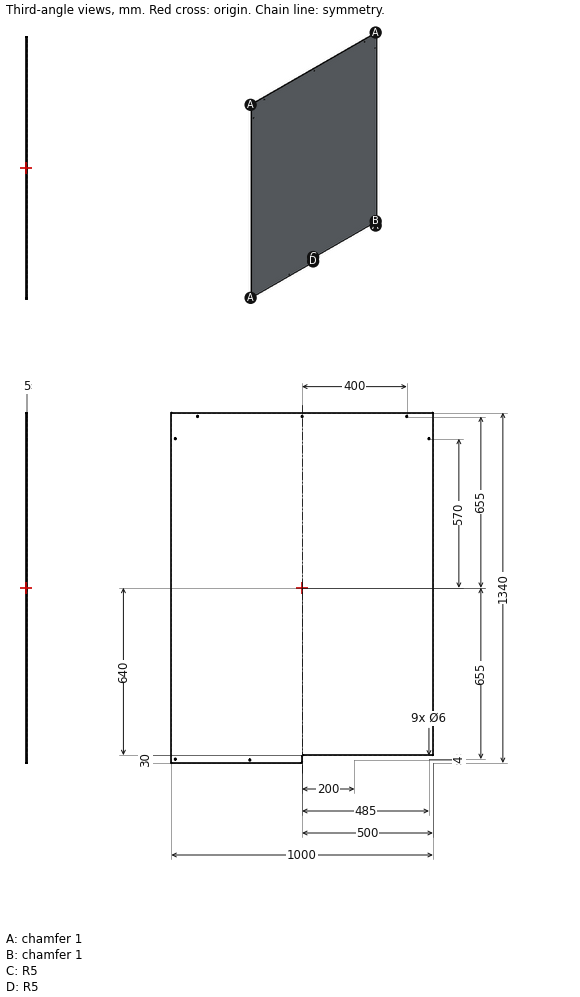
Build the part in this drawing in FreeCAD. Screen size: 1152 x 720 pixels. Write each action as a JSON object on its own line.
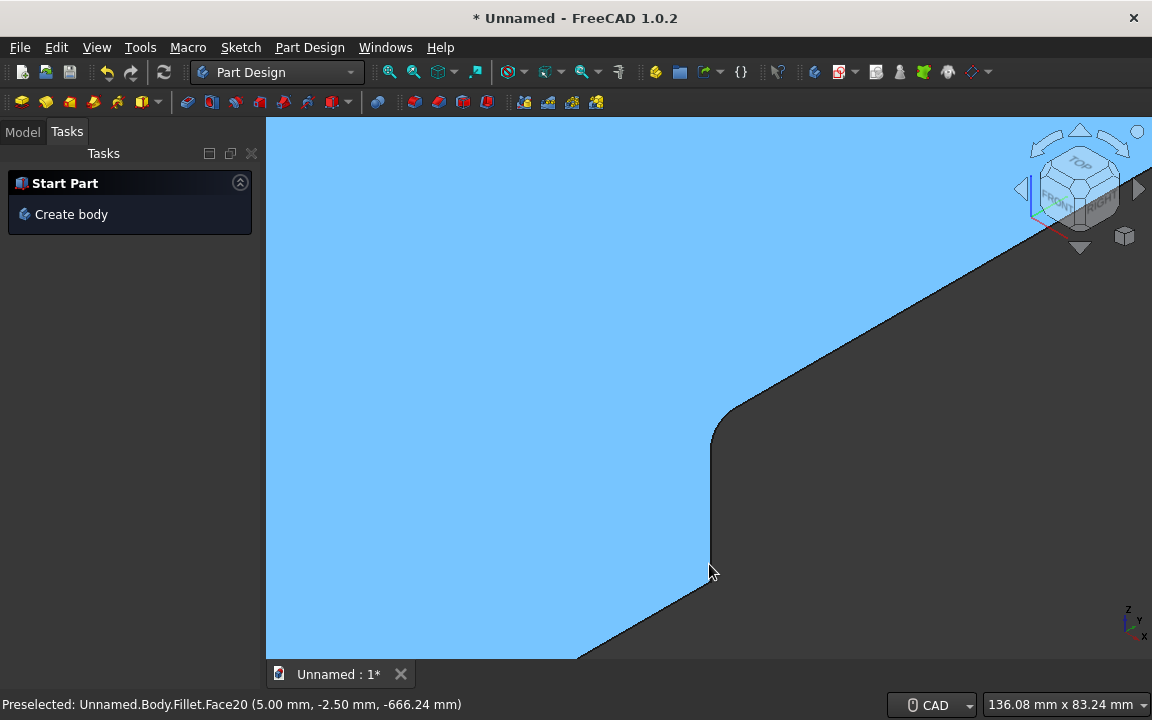
{"action": "left_click", "coordinate": [390, 72]}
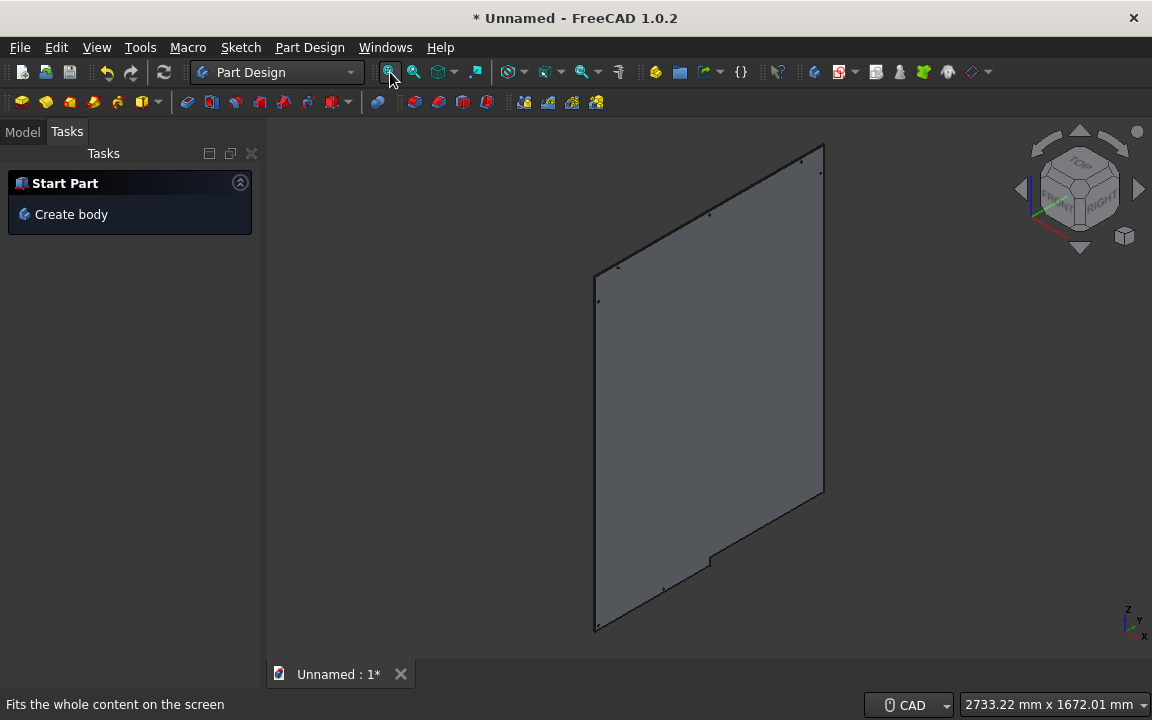
{"action": "key", "text": "1"}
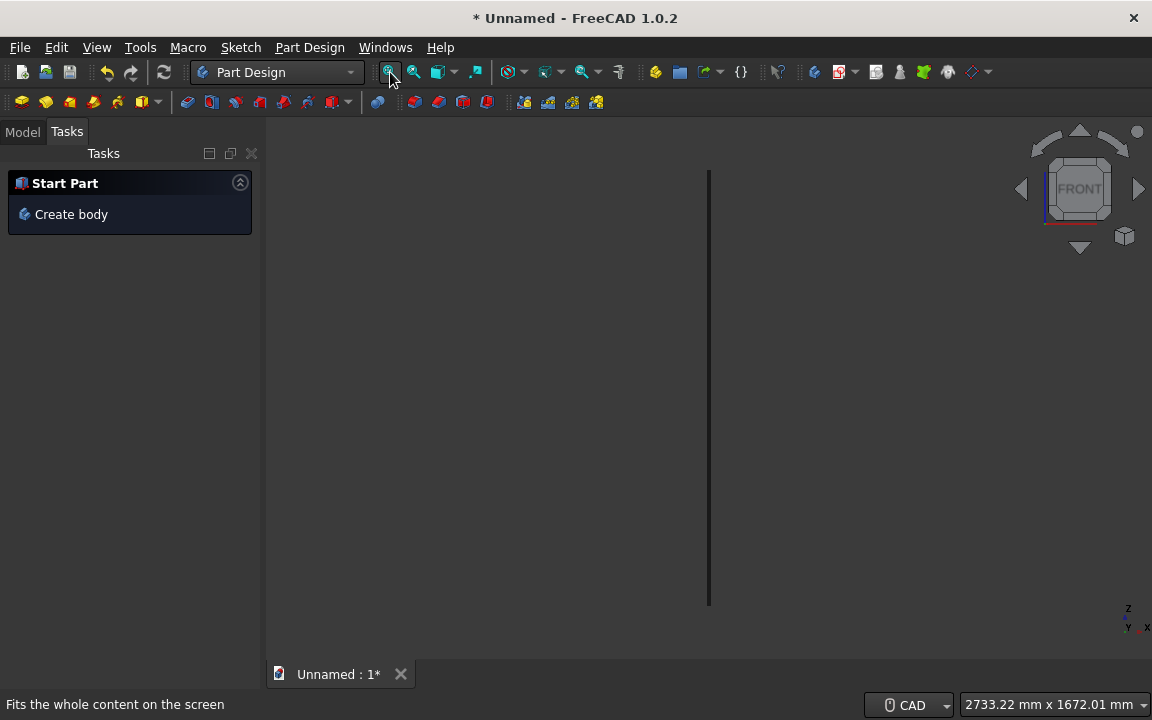
{"action": "scroll", "coordinate": [709, 604], "scroll_direction": "up", "scroll_amount": 15}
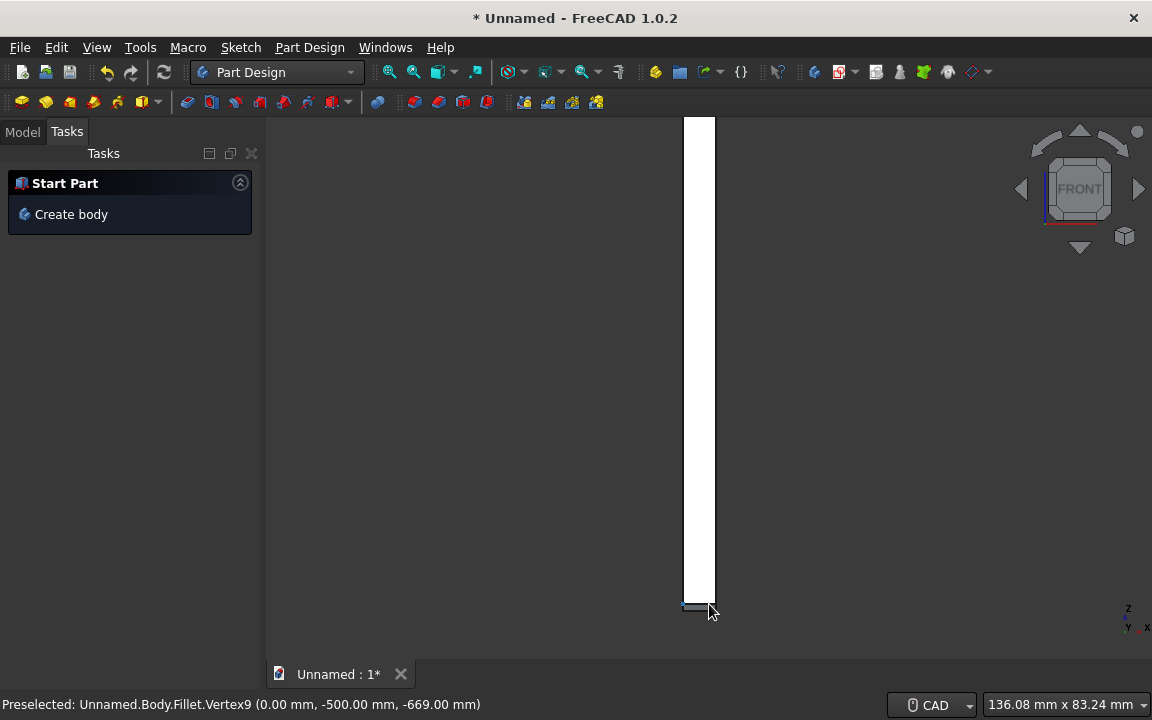
{"action": "left_click", "coordinate": [390, 72]}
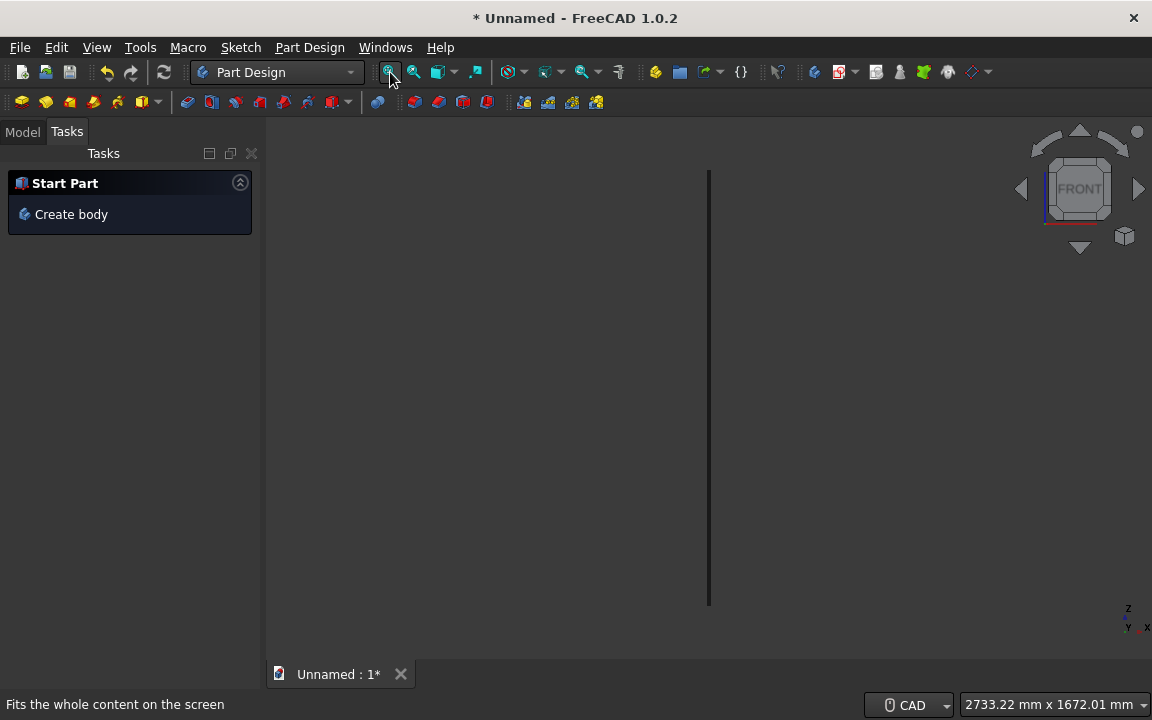
{"action": "key", "text": "3"}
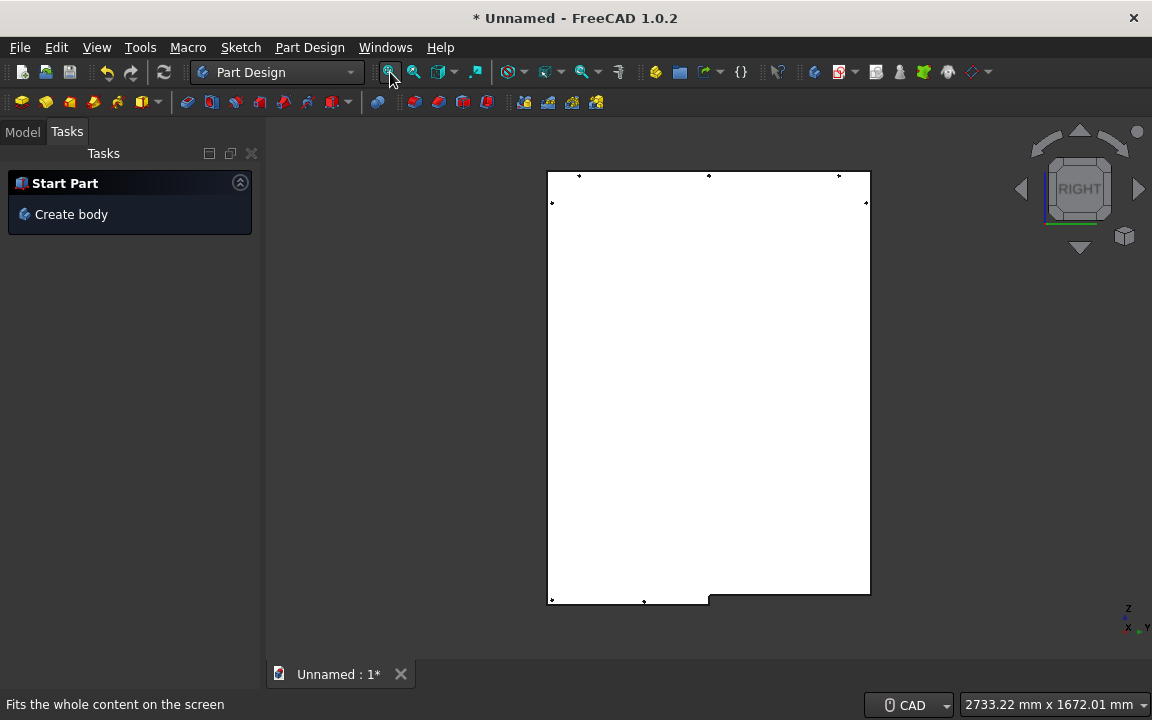
{"action": "scroll", "coordinate": [709, 604], "scroll_direction": "up", "scroll_amount": 15}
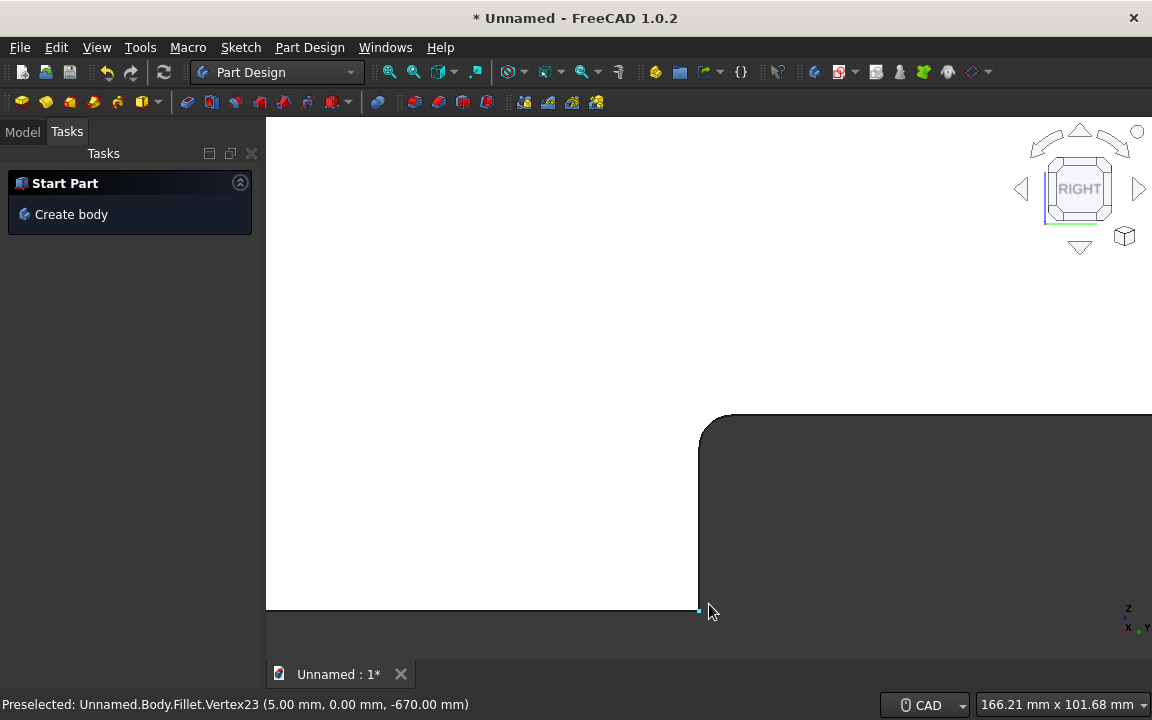
{"action": "left_click", "coordinate": [390, 72]}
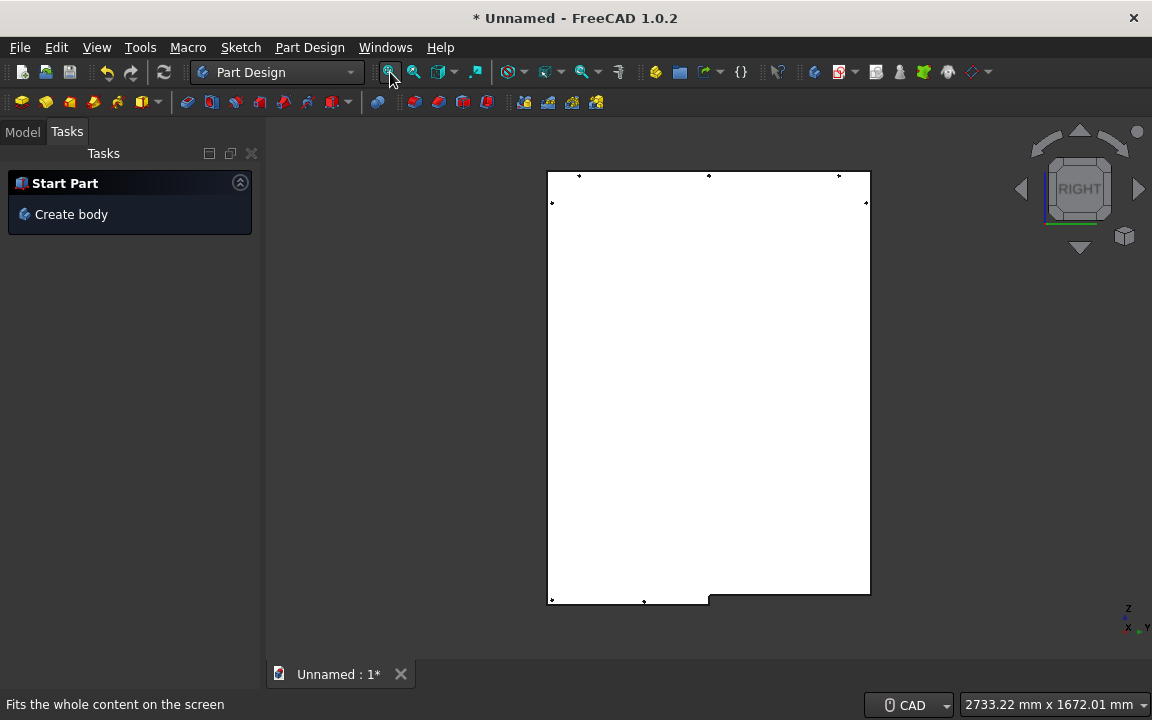
{"action": "key", "text": "5"}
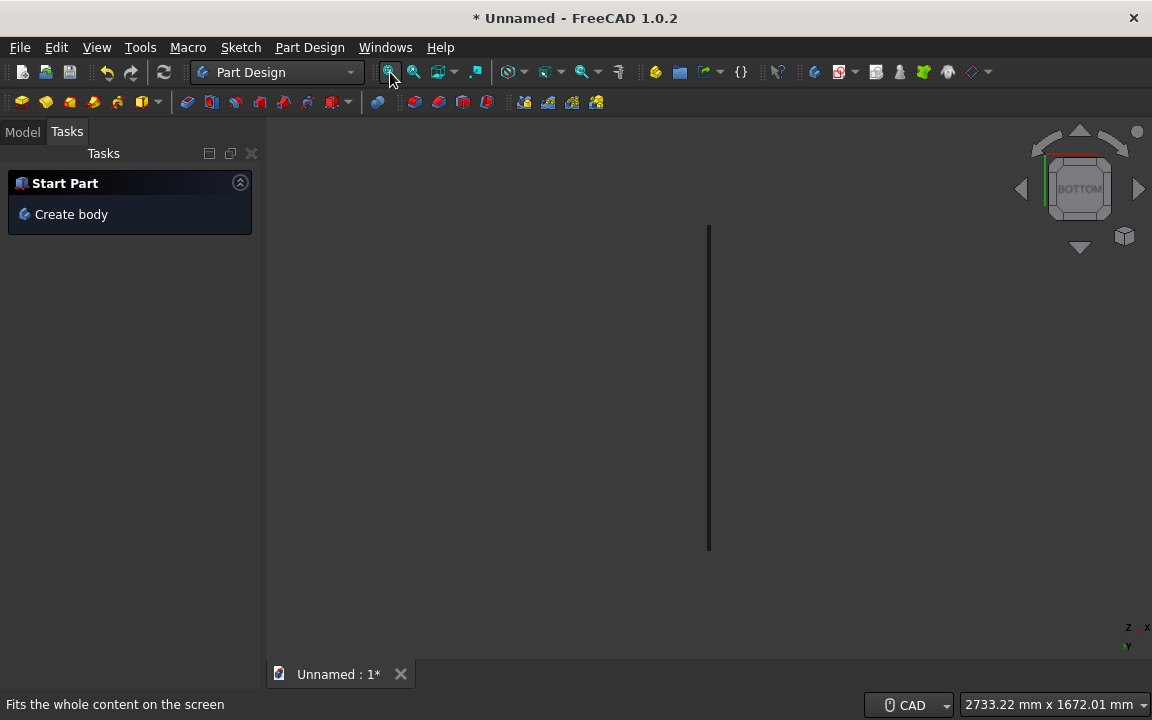
{"action": "scroll", "coordinate": [709, 387], "scroll_direction": "up", "scroll_amount": 15}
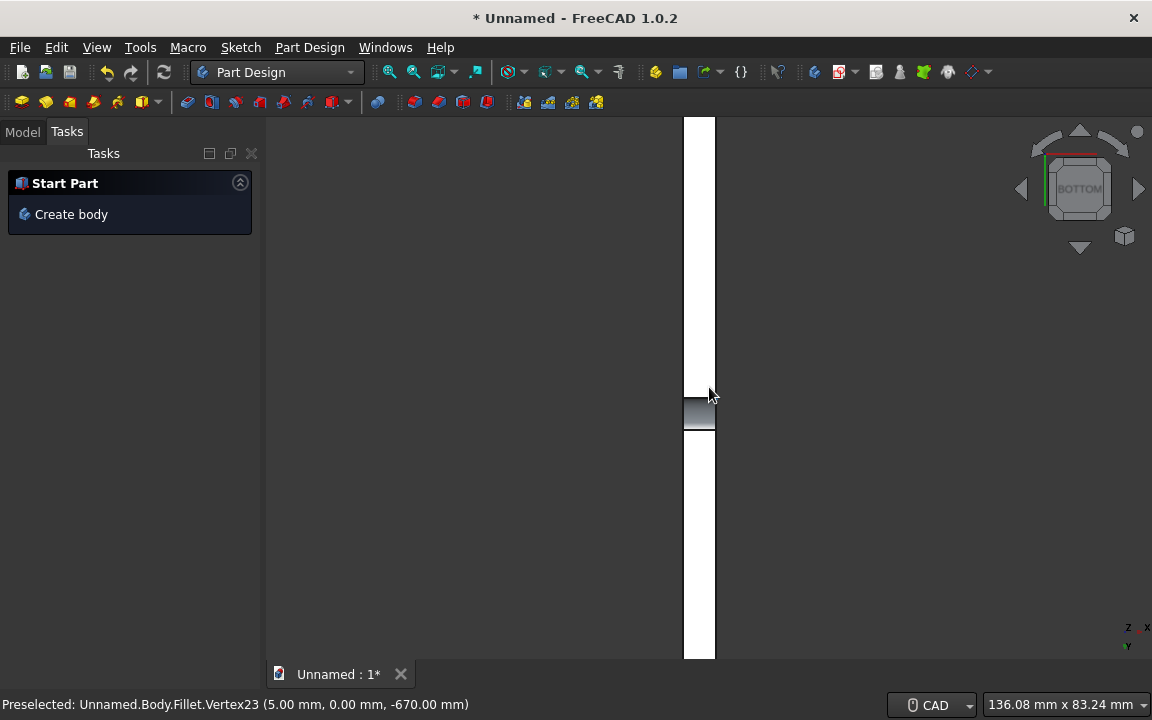
{"action": "left_click", "coordinate": [699, 397]}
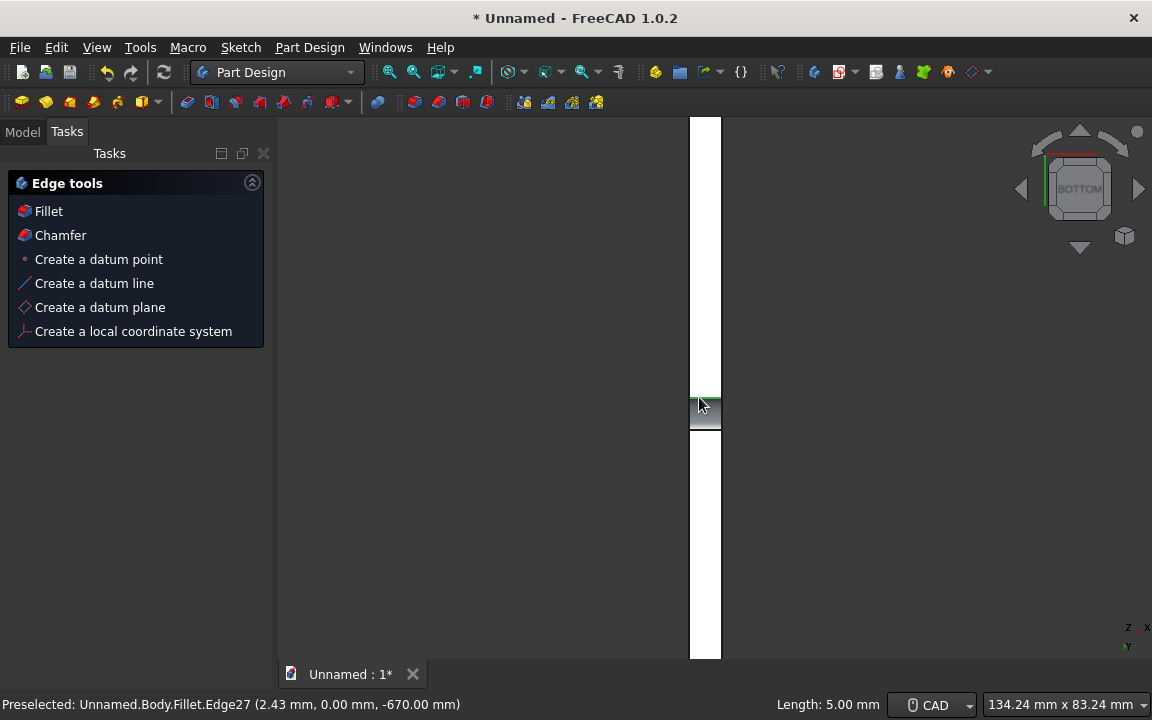
{"action": "left_click", "coordinate": [416, 102]}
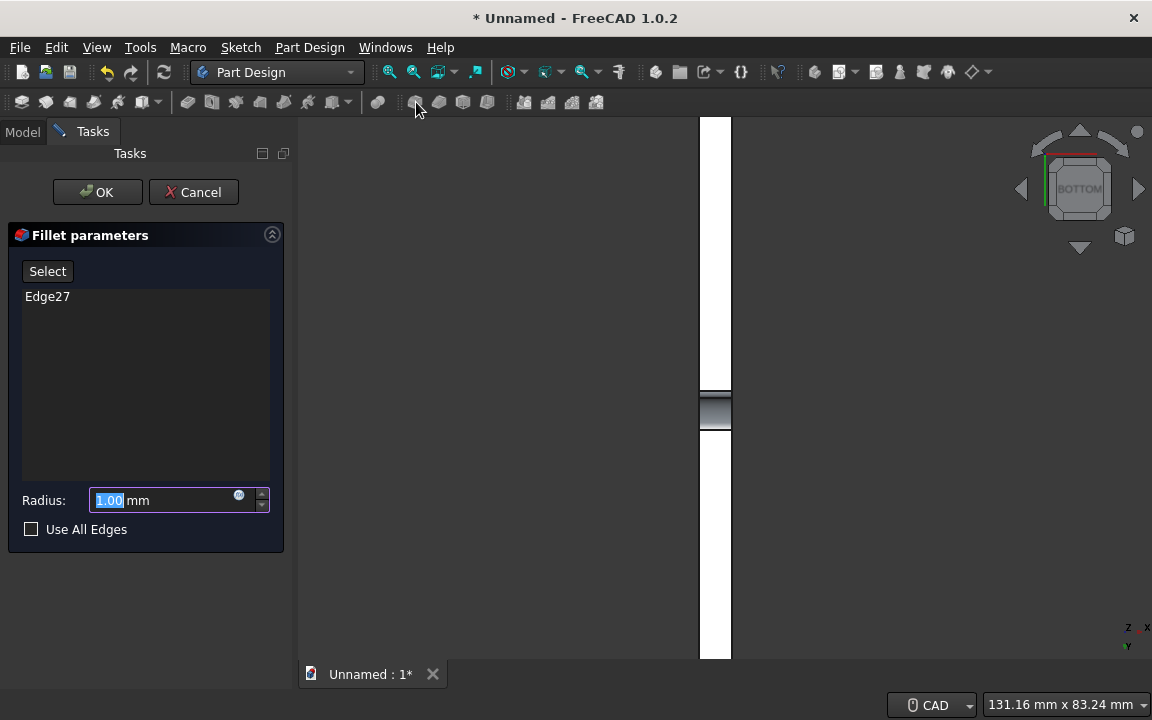
{"action": "type", "text": "5"}
{"action": "key", "text": "Tab"}